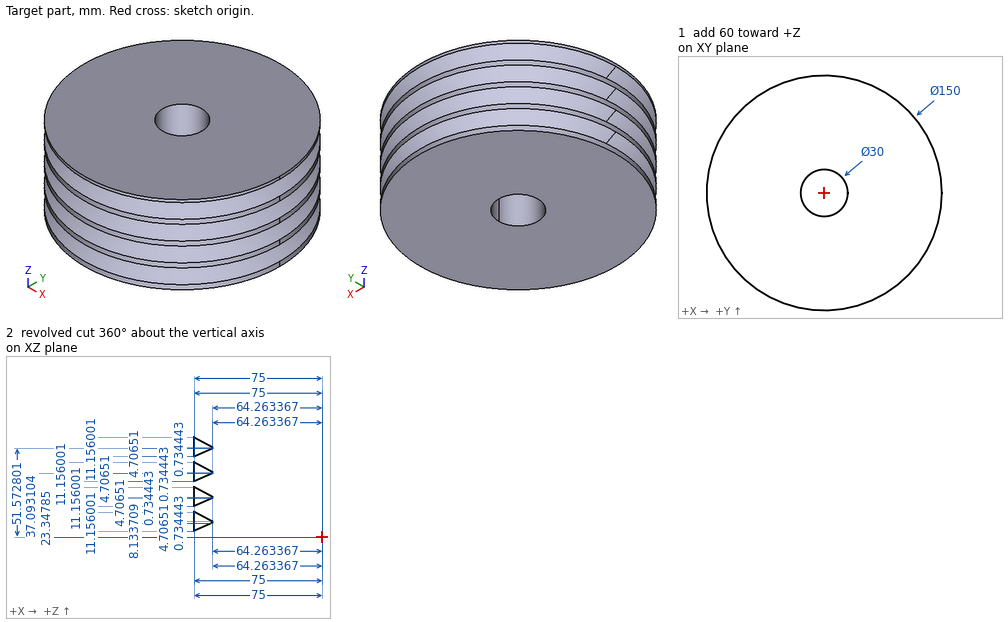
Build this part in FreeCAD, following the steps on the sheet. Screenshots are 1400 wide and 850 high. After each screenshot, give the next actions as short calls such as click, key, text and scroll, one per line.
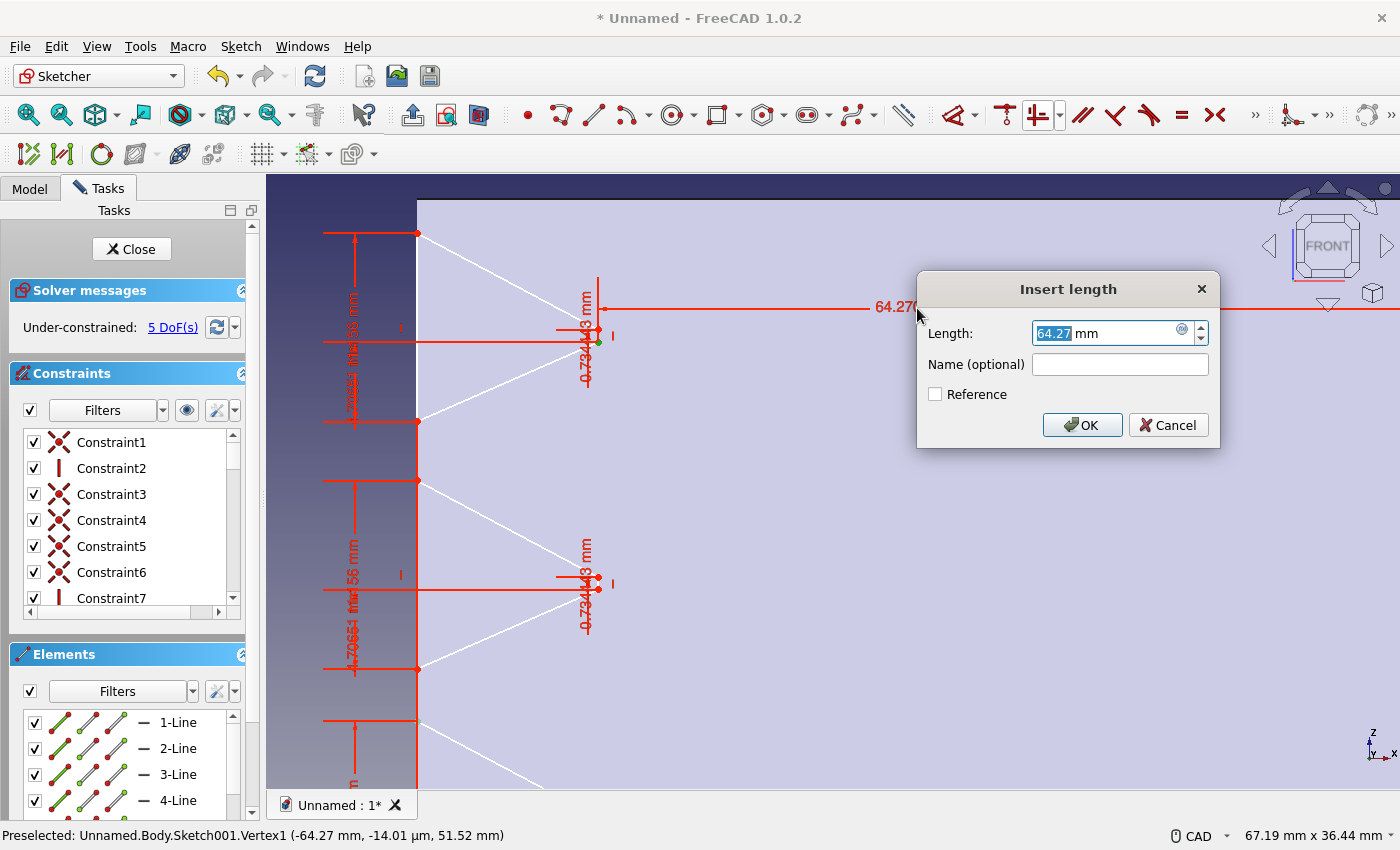
text(64.263367)
key(Return)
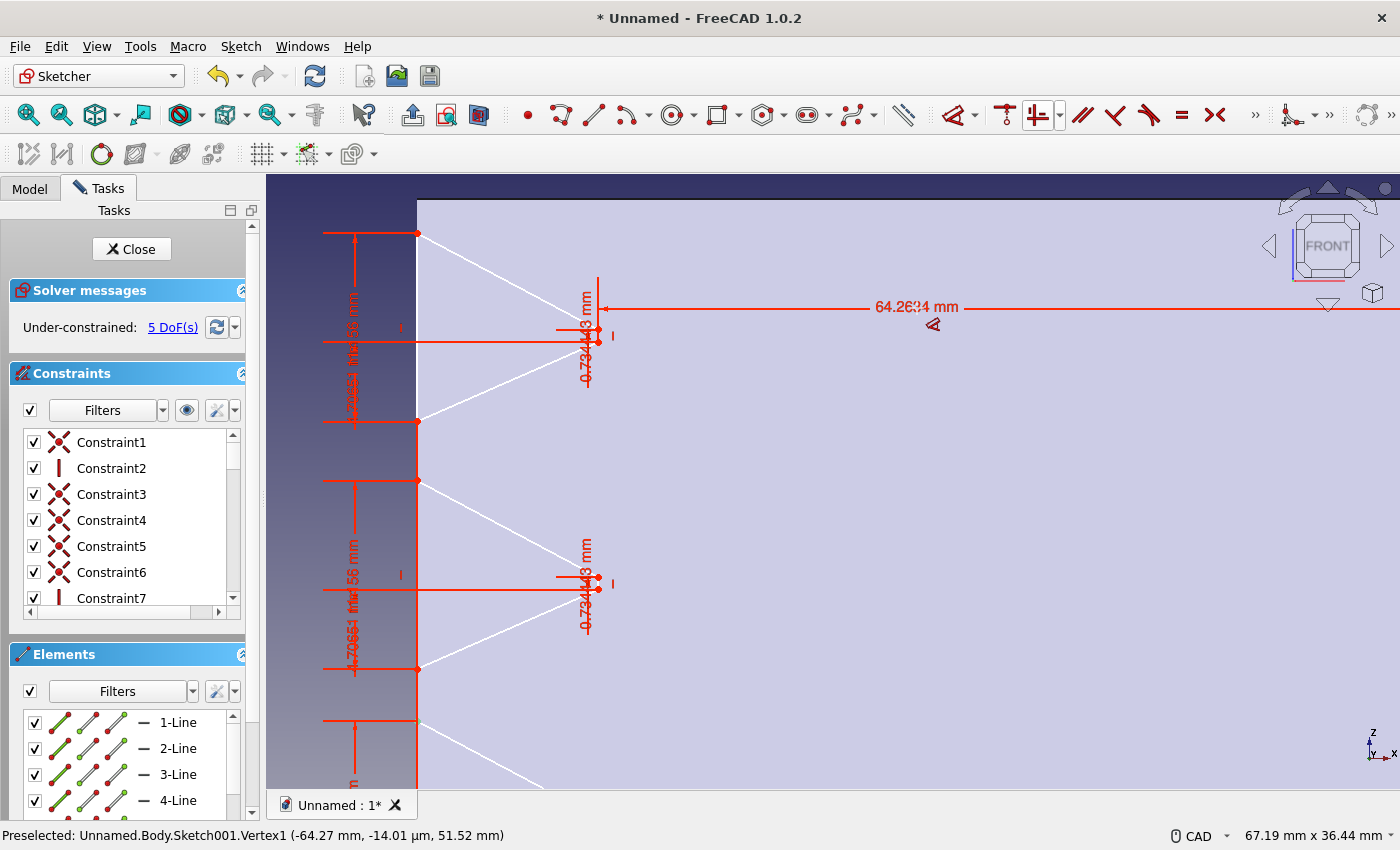
click(598, 342)
click(564, 455)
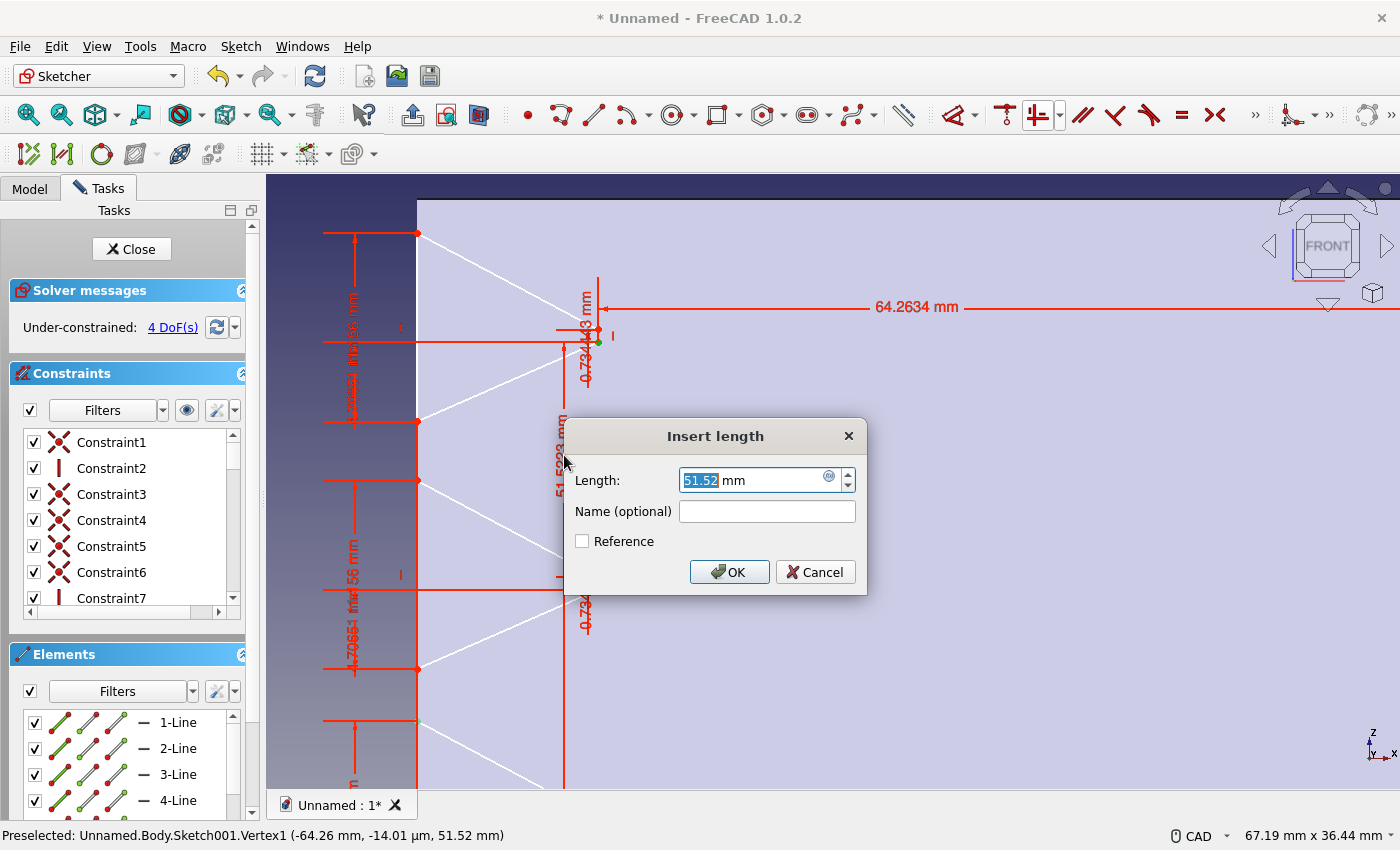
text(51.572801)
key(Return)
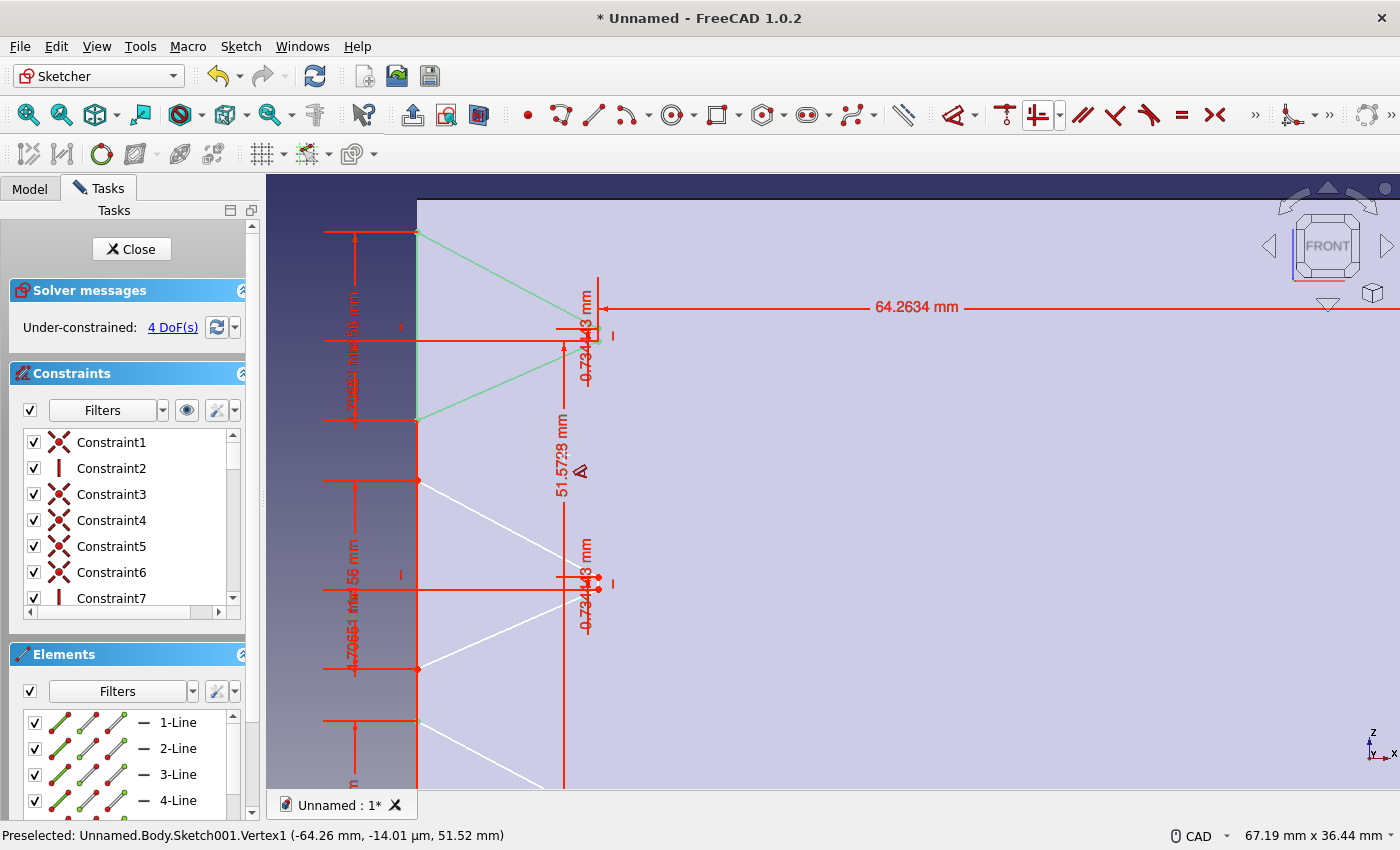
click(598, 590)
click(917, 556)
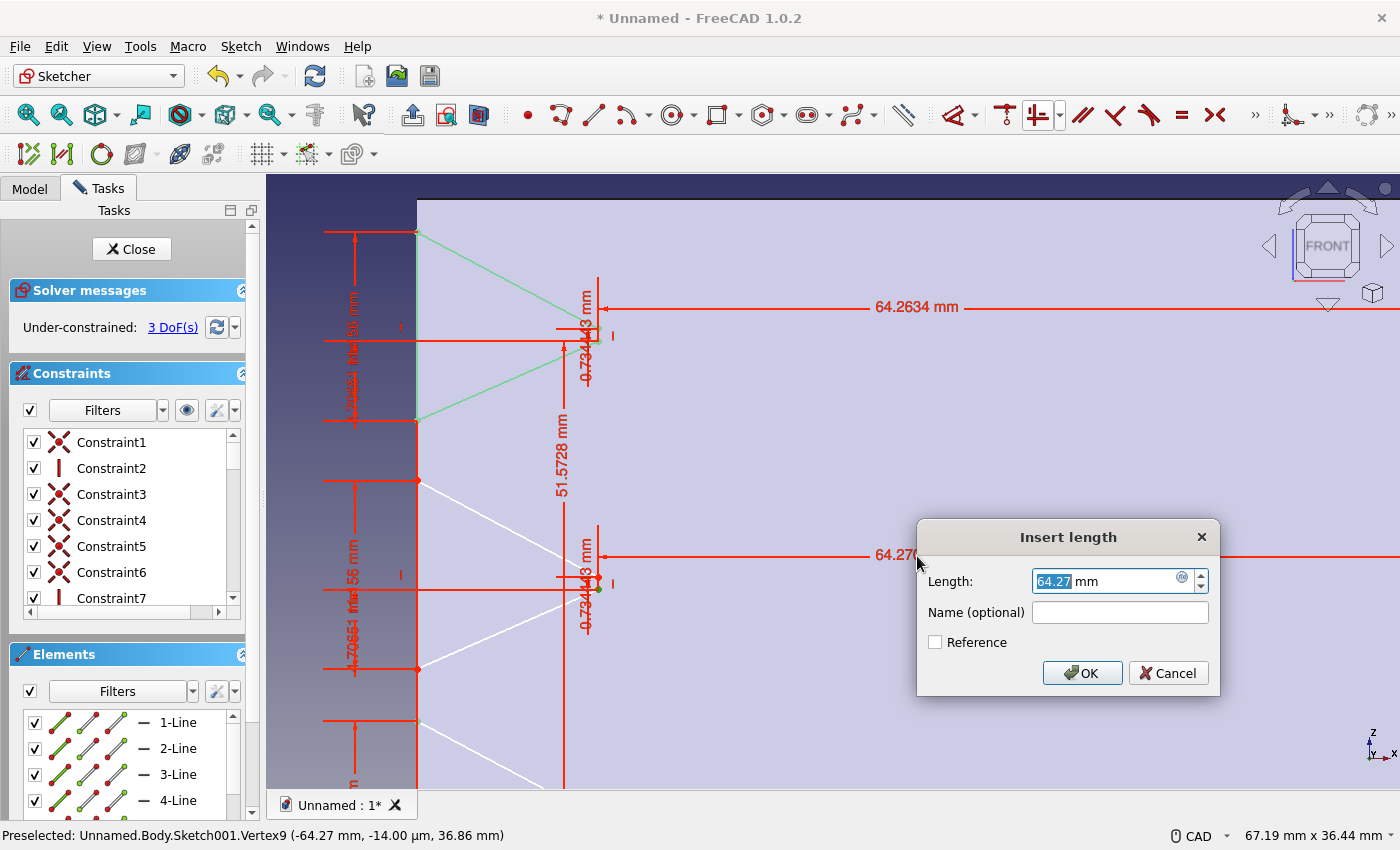
text(64.263367)
key(Return)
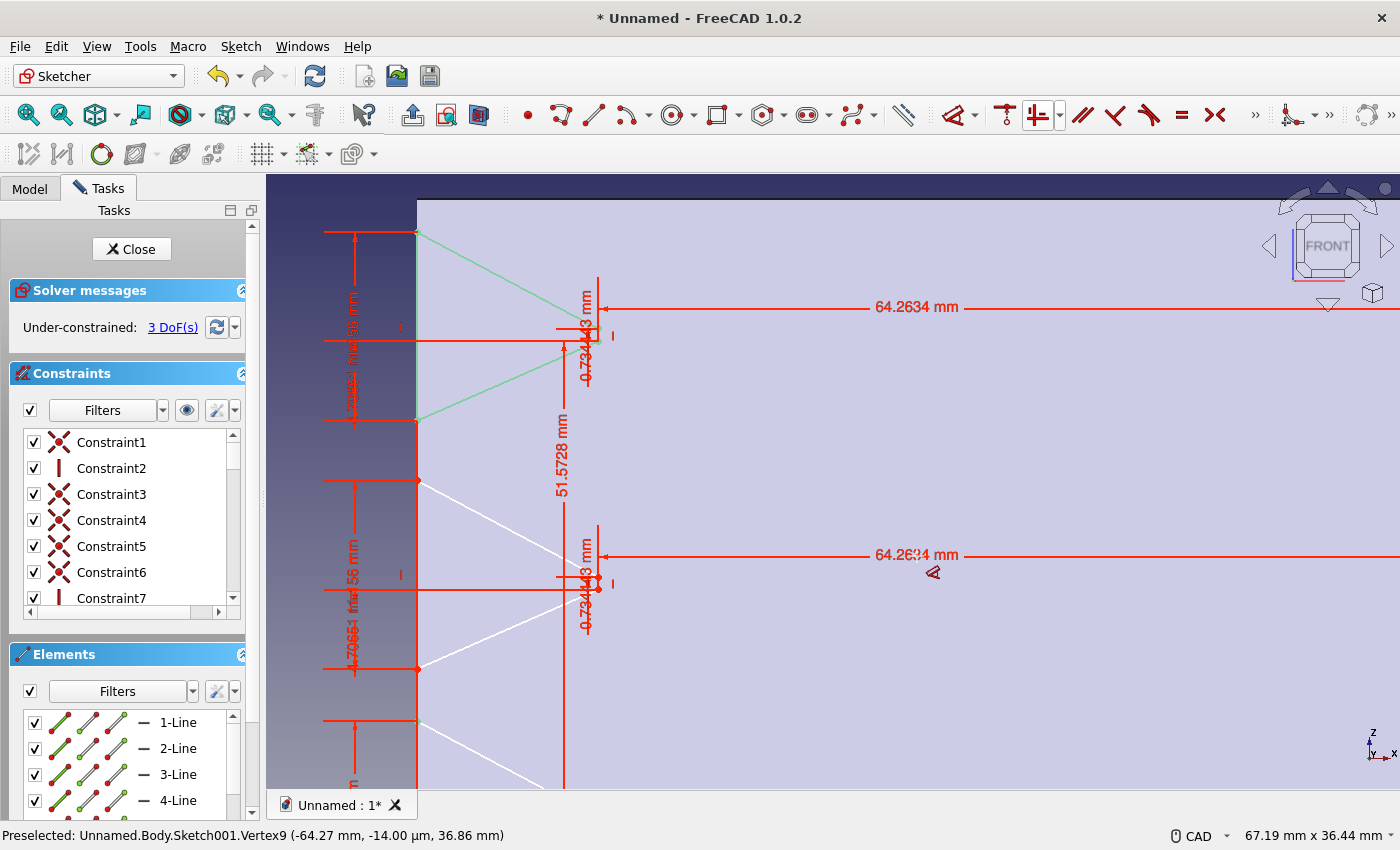
click(598, 590)
click(564, 675)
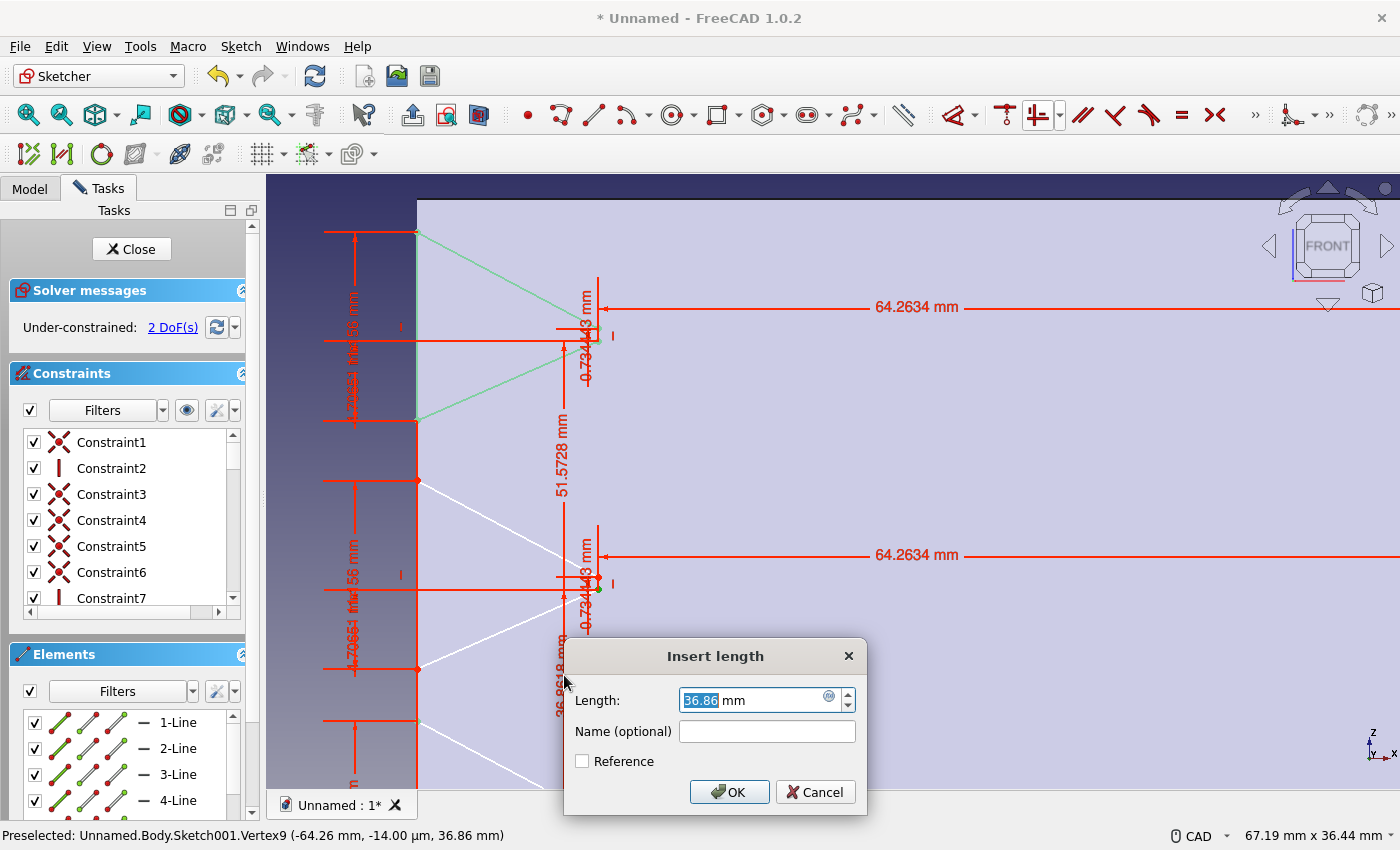
text(37.093104)
key(Return)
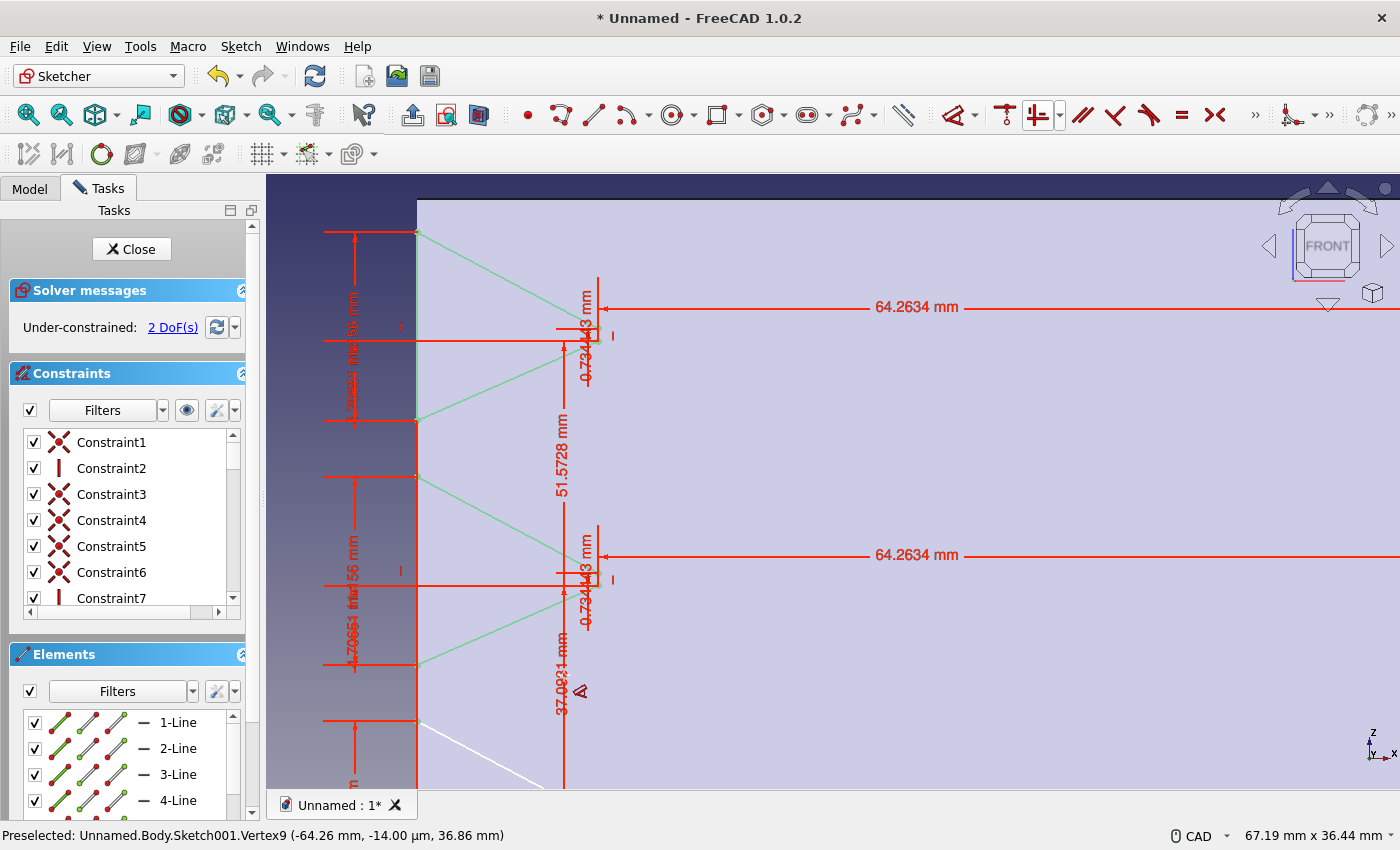
scroll(598, 341, down, 5)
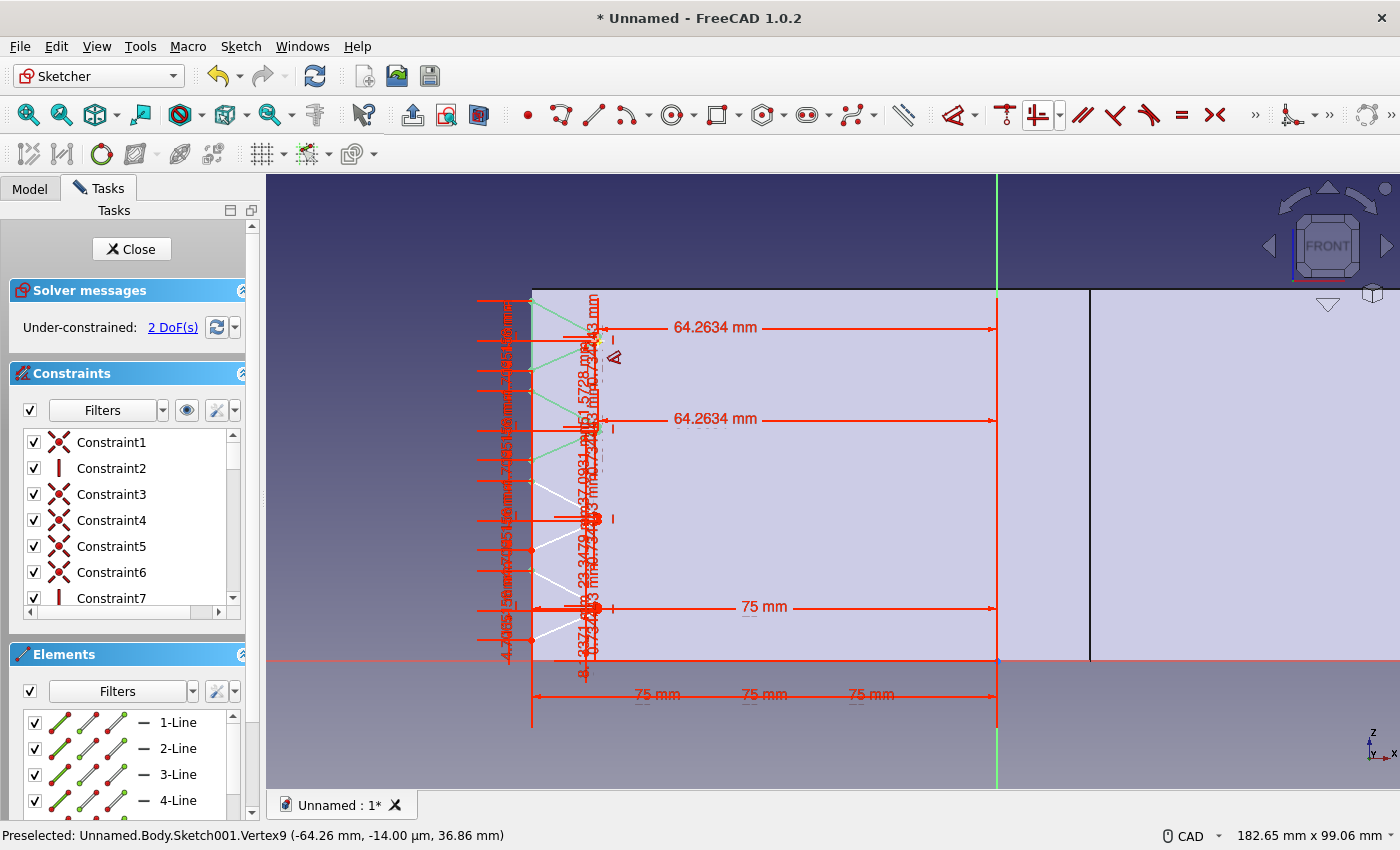
scroll(598, 521, up, 5)